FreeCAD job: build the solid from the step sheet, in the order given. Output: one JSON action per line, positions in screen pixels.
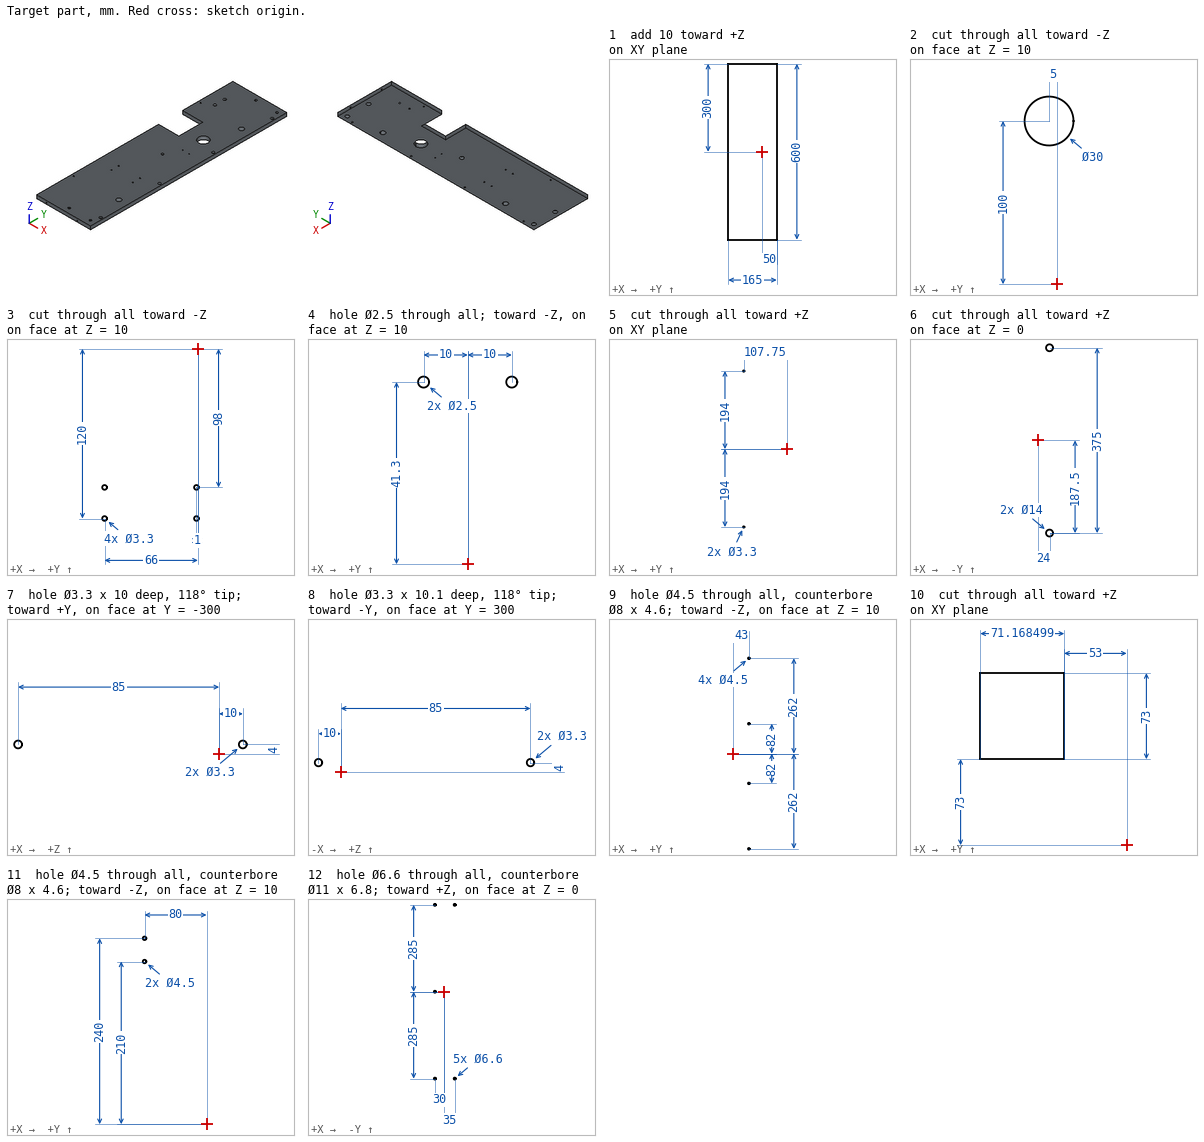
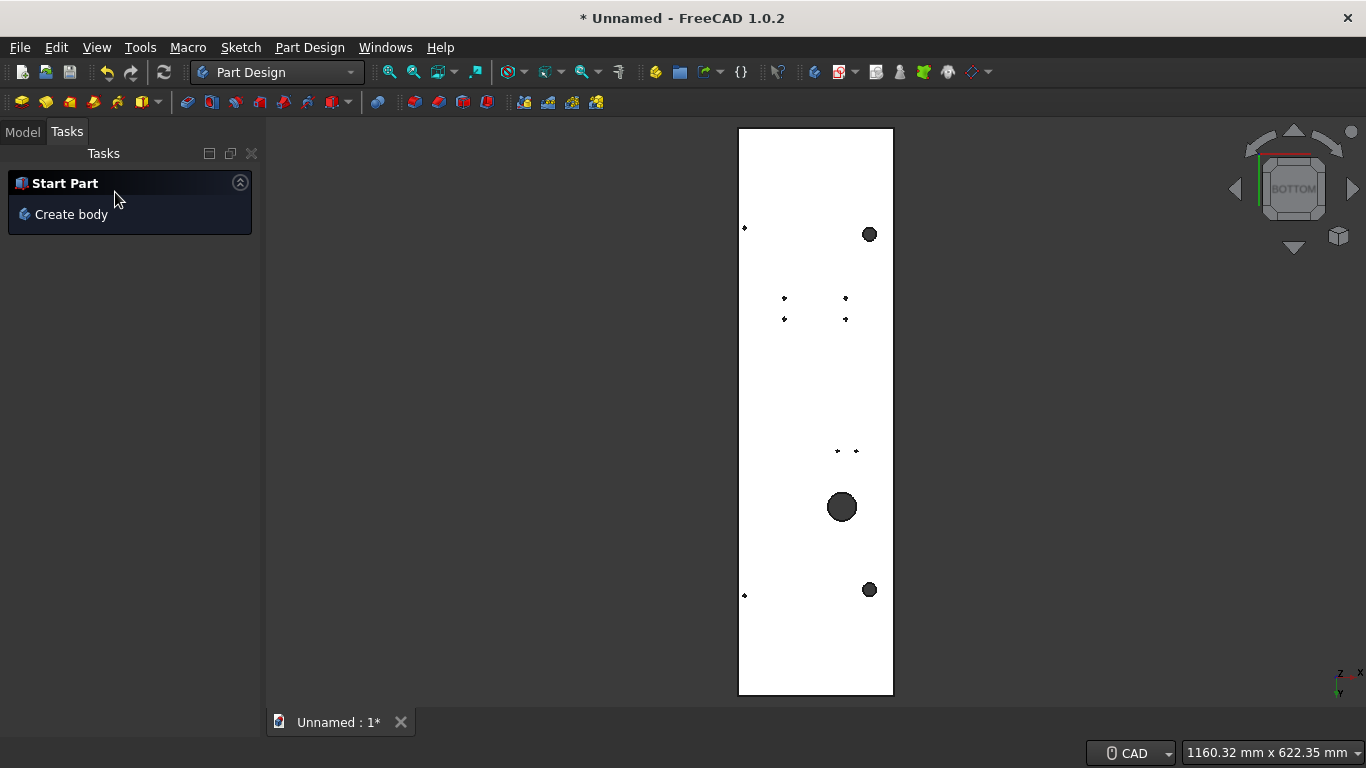
{"action": "key", "text": "0"}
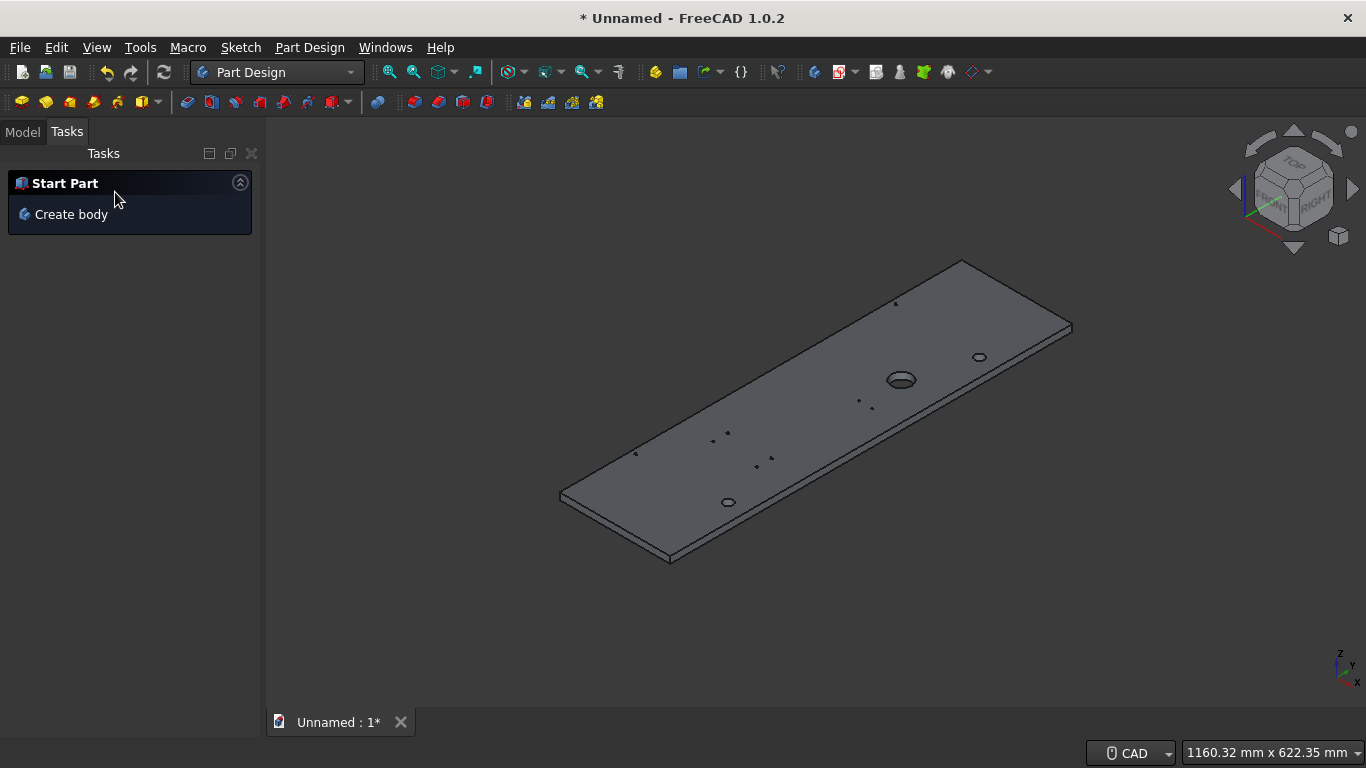
{"action": "scroll", "coordinate": [662, 554], "scroll_direction": "up", "scroll_amount": 5}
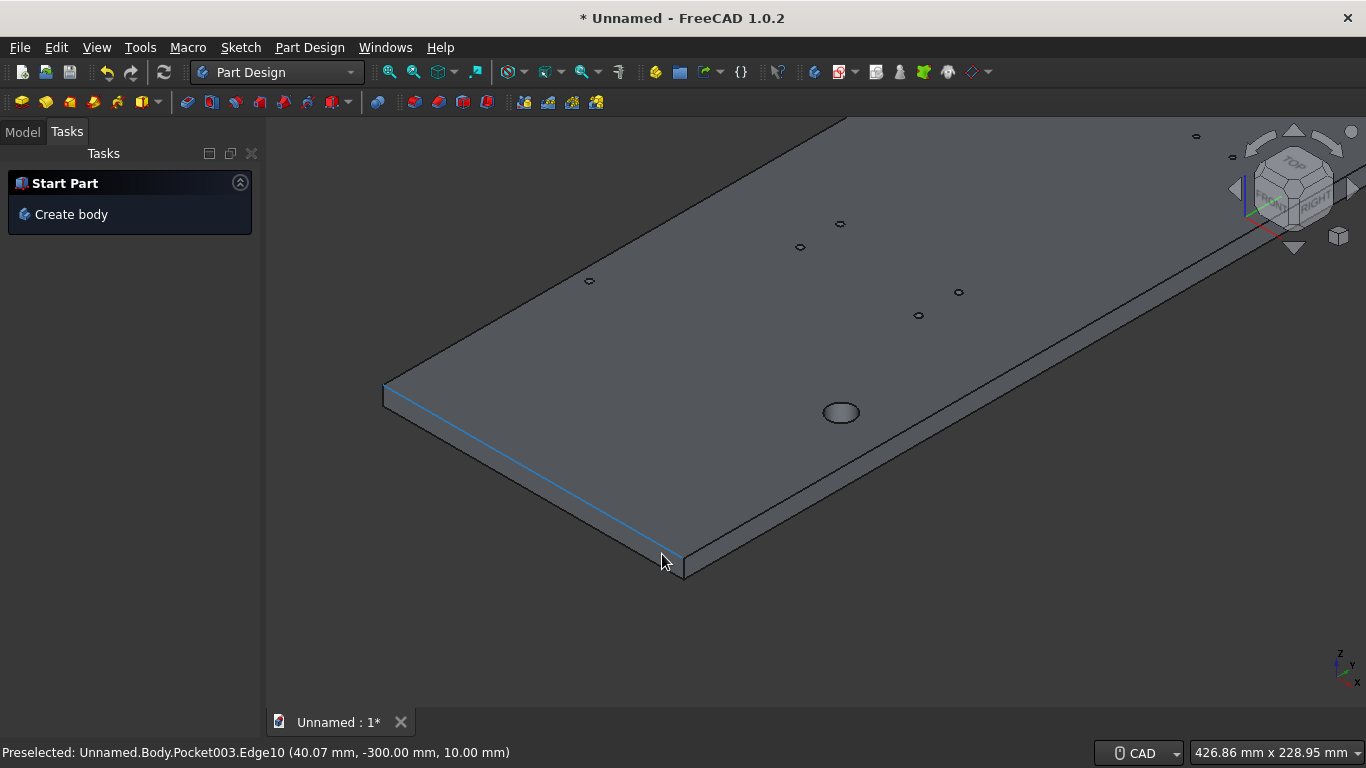
{"action": "left_click", "coordinate": [662, 556]}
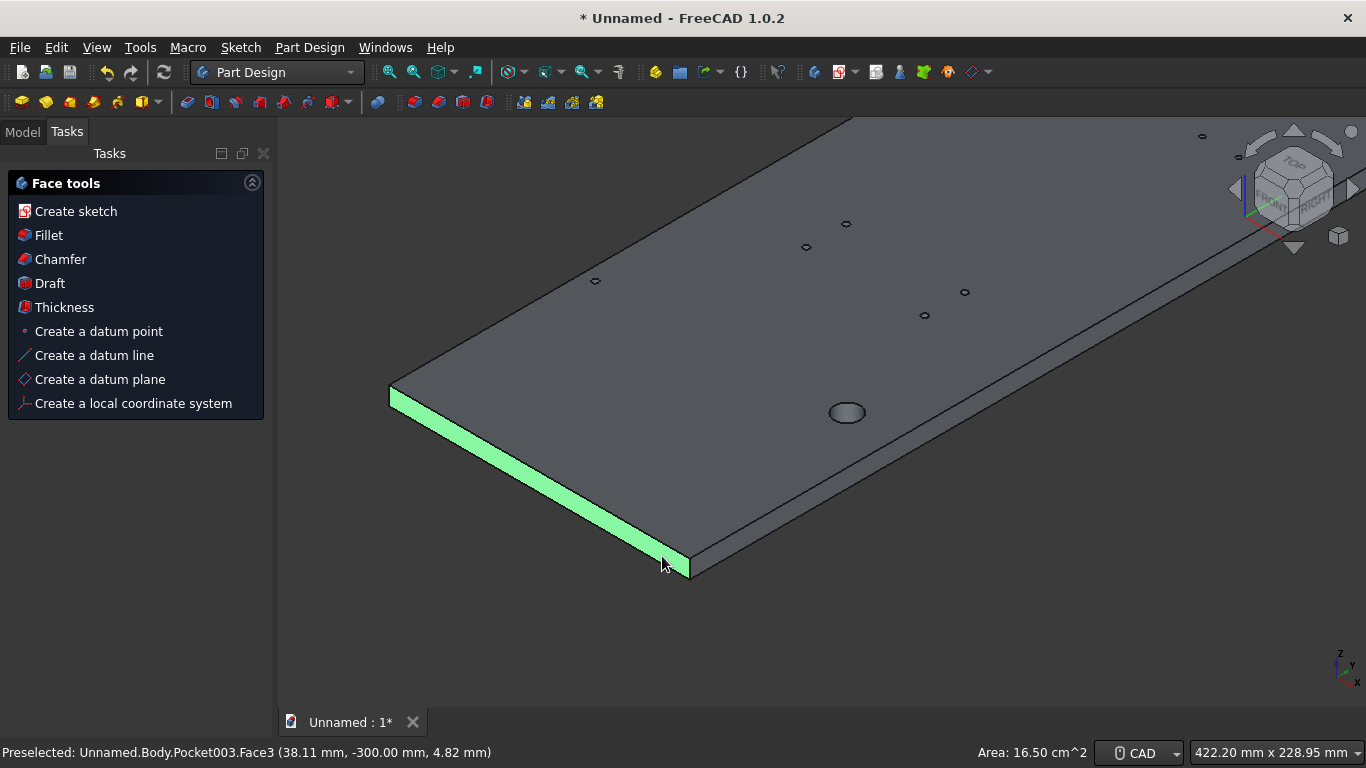
{"action": "left_click", "coordinate": [840, 72]}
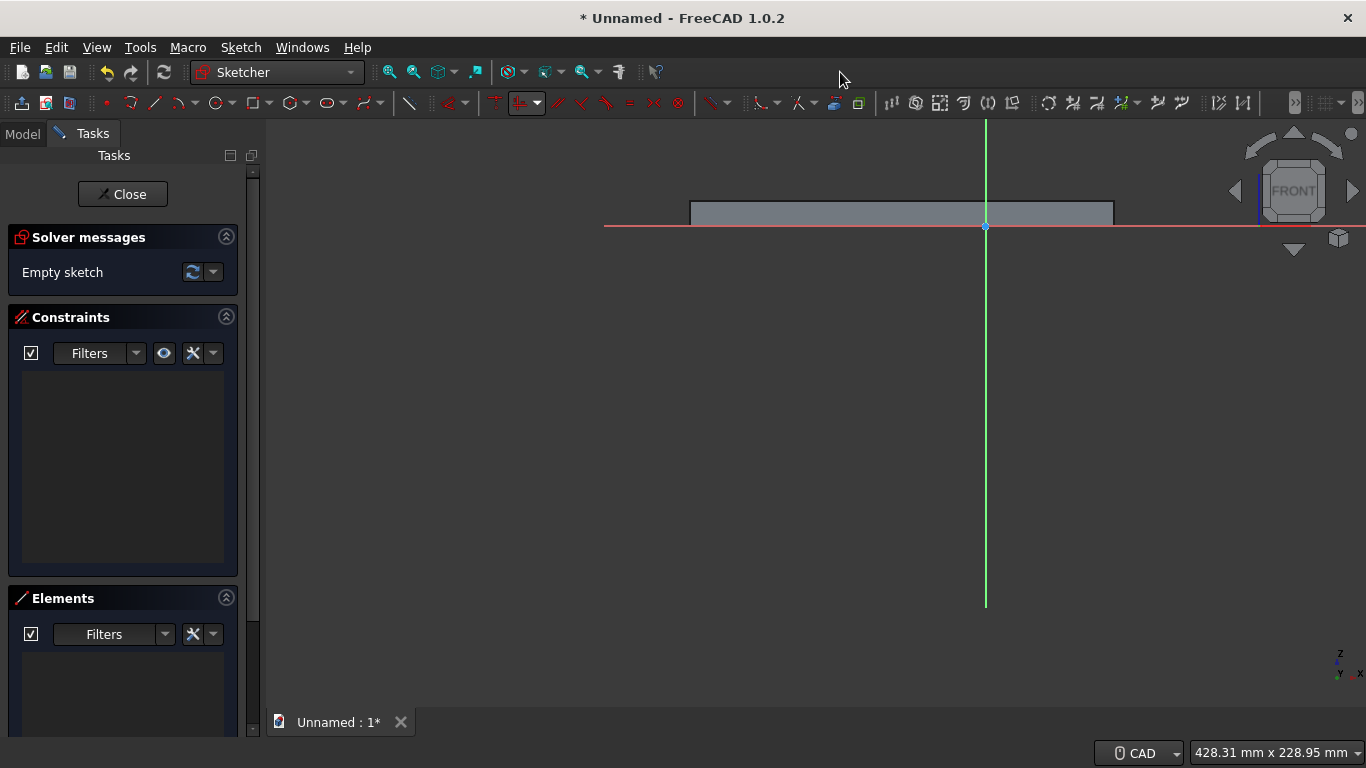
{"action": "scroll", "coordinate": [972, 147], "scroll_direction": "up", "scroll_amount": 5}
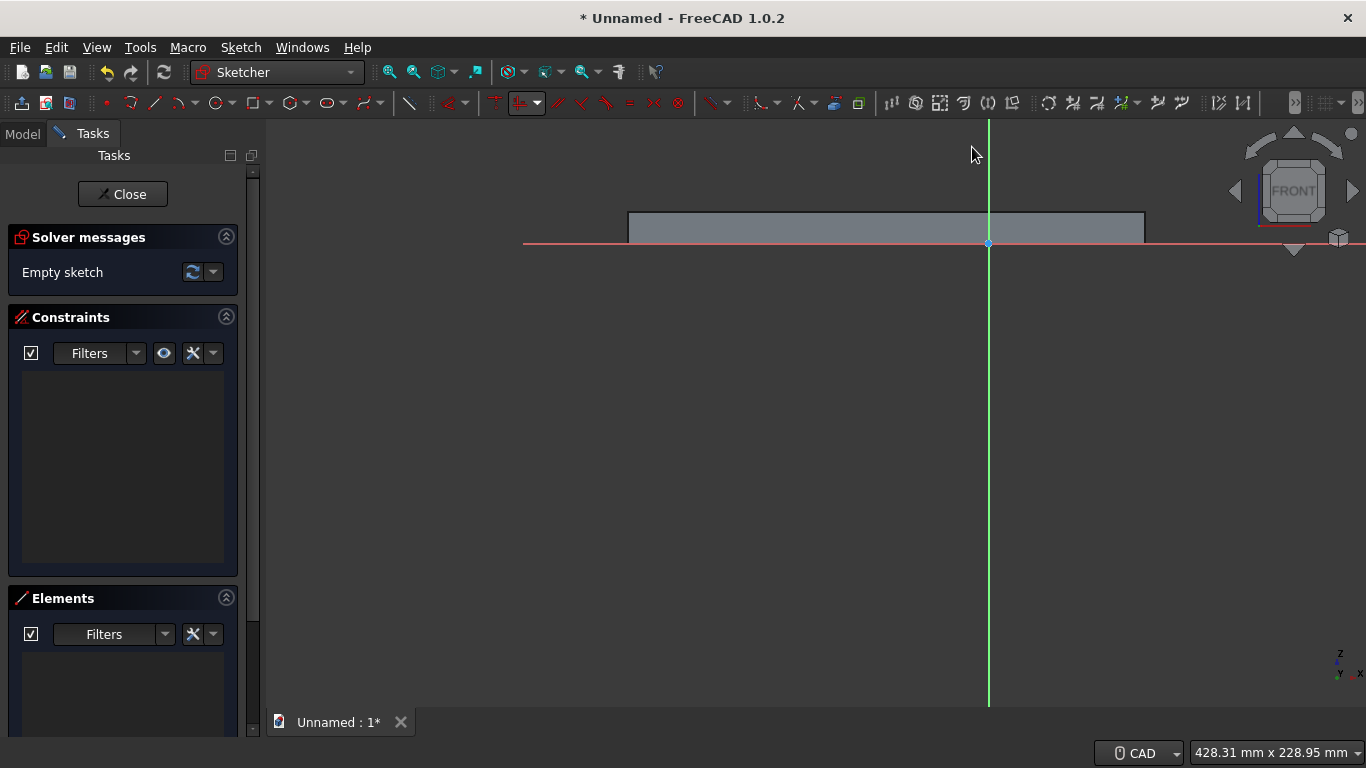
{"action": "left_click", "coordinate": [216, 104]}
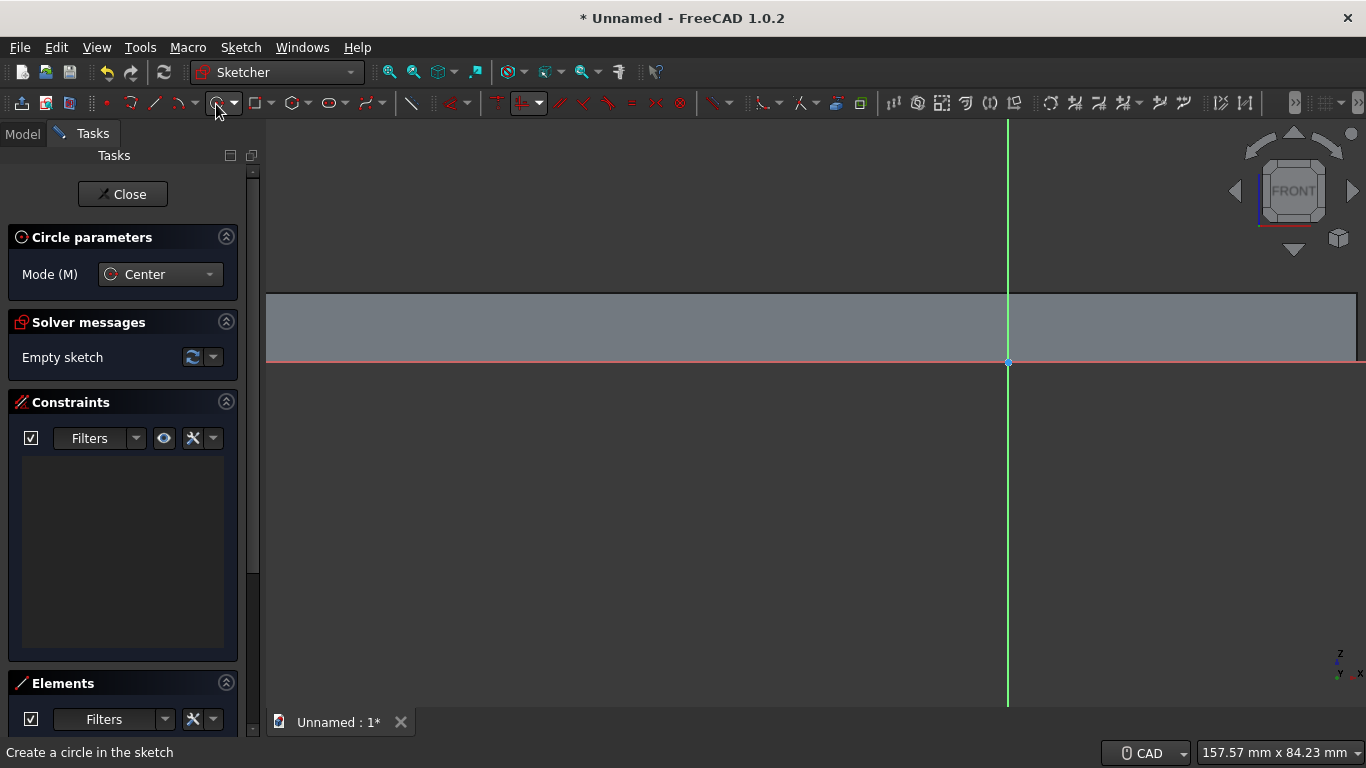
{"action": "scroll", "coordinate": [1078, 334], "scroll_direction": "up", "scroll_amount": 4}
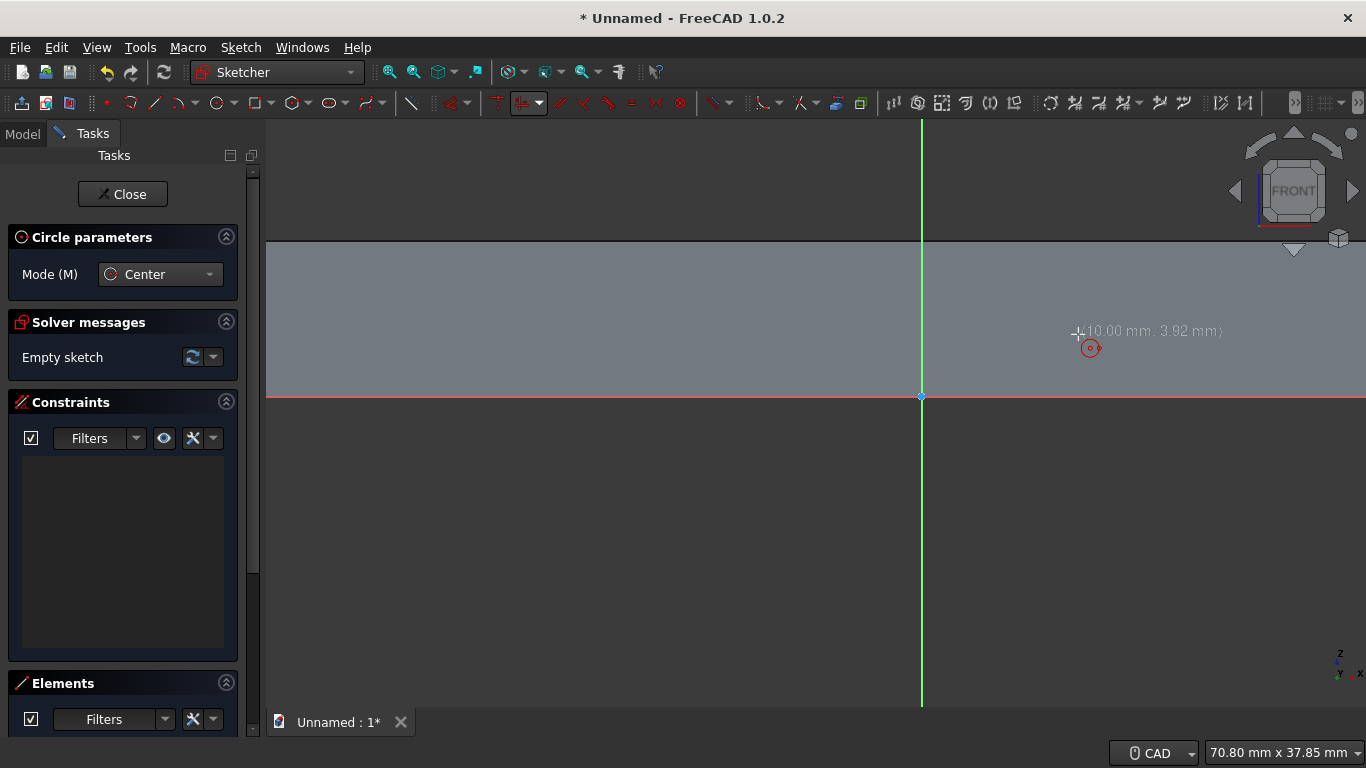
{"action": "left_click", "coordinate": [1077, 335]}
{"action": "mouse_move", "coordinate": [1095, 316]}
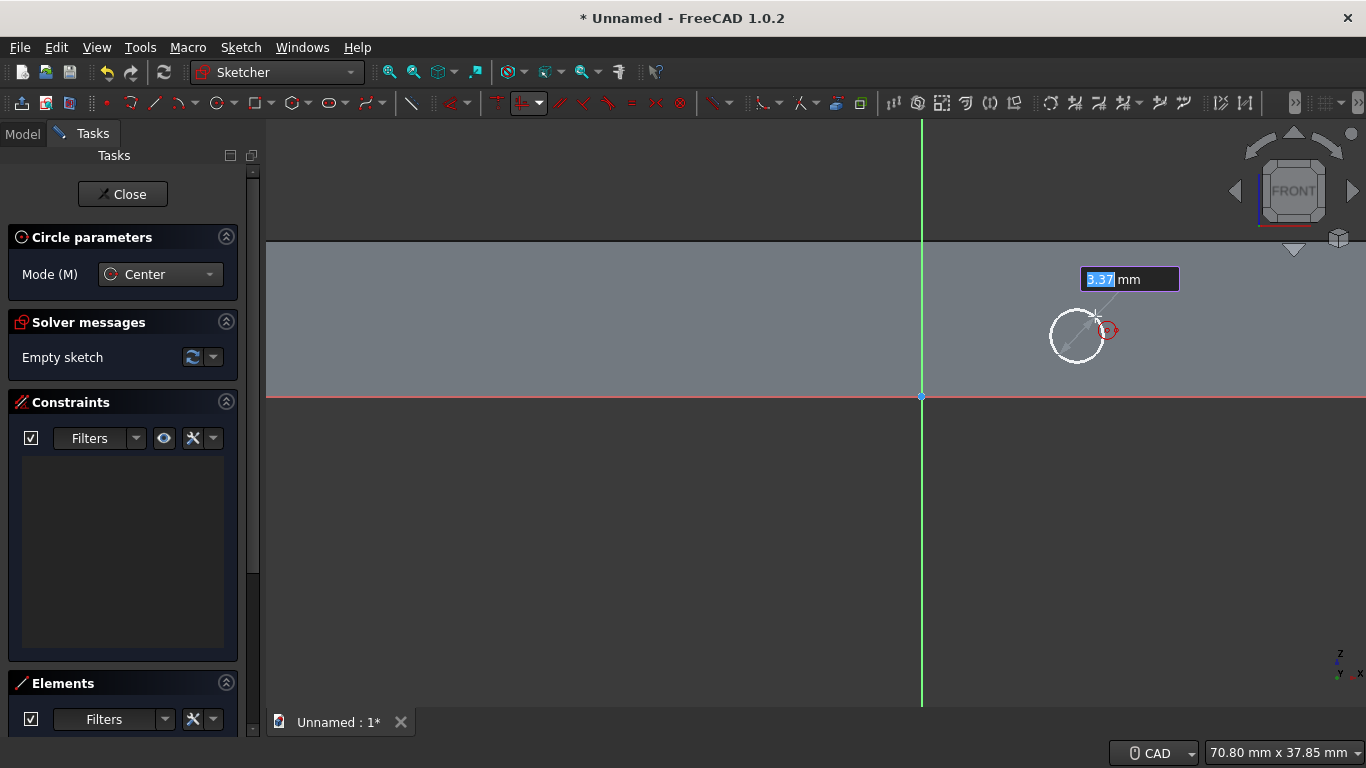
{"action": "type", "text": "3.3"}
{"action": "key", "text": "Return"}